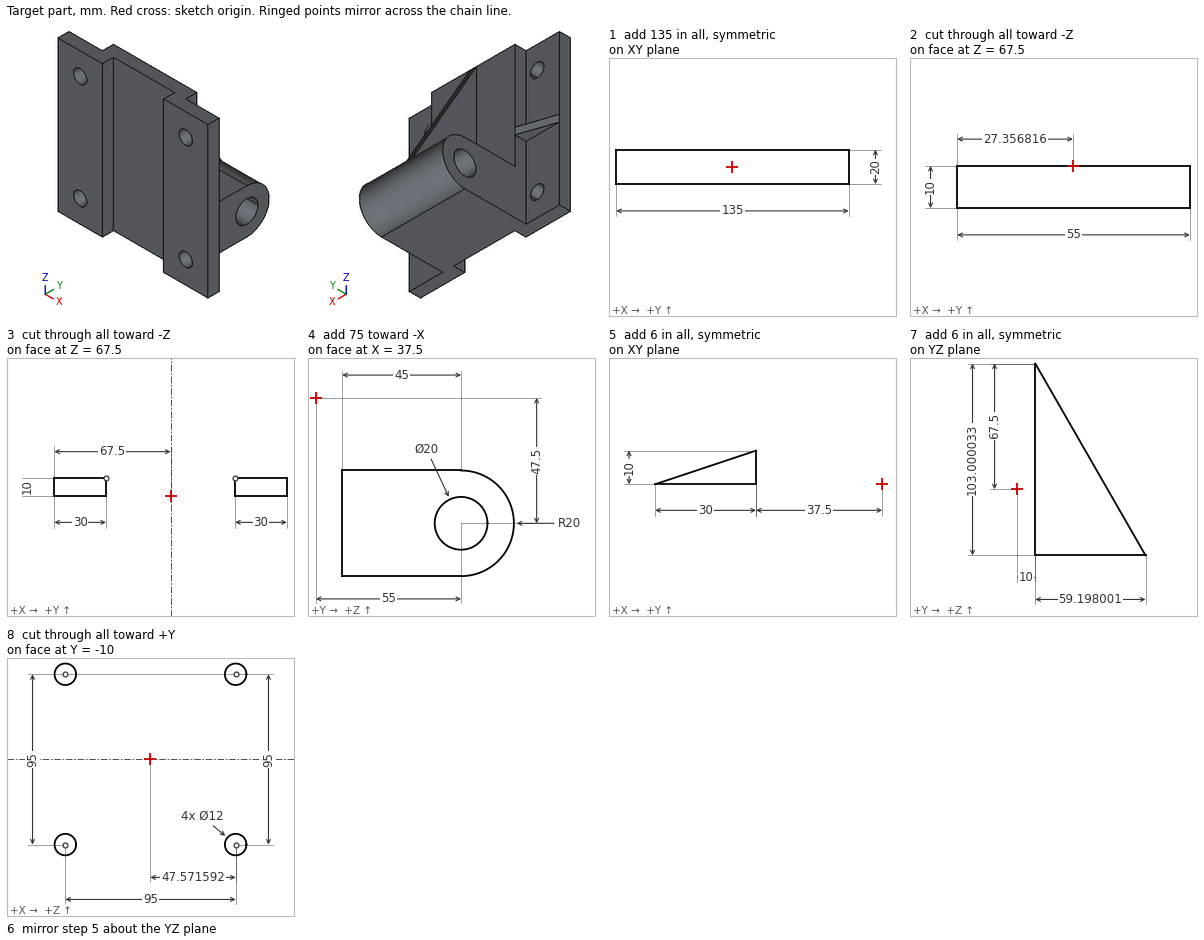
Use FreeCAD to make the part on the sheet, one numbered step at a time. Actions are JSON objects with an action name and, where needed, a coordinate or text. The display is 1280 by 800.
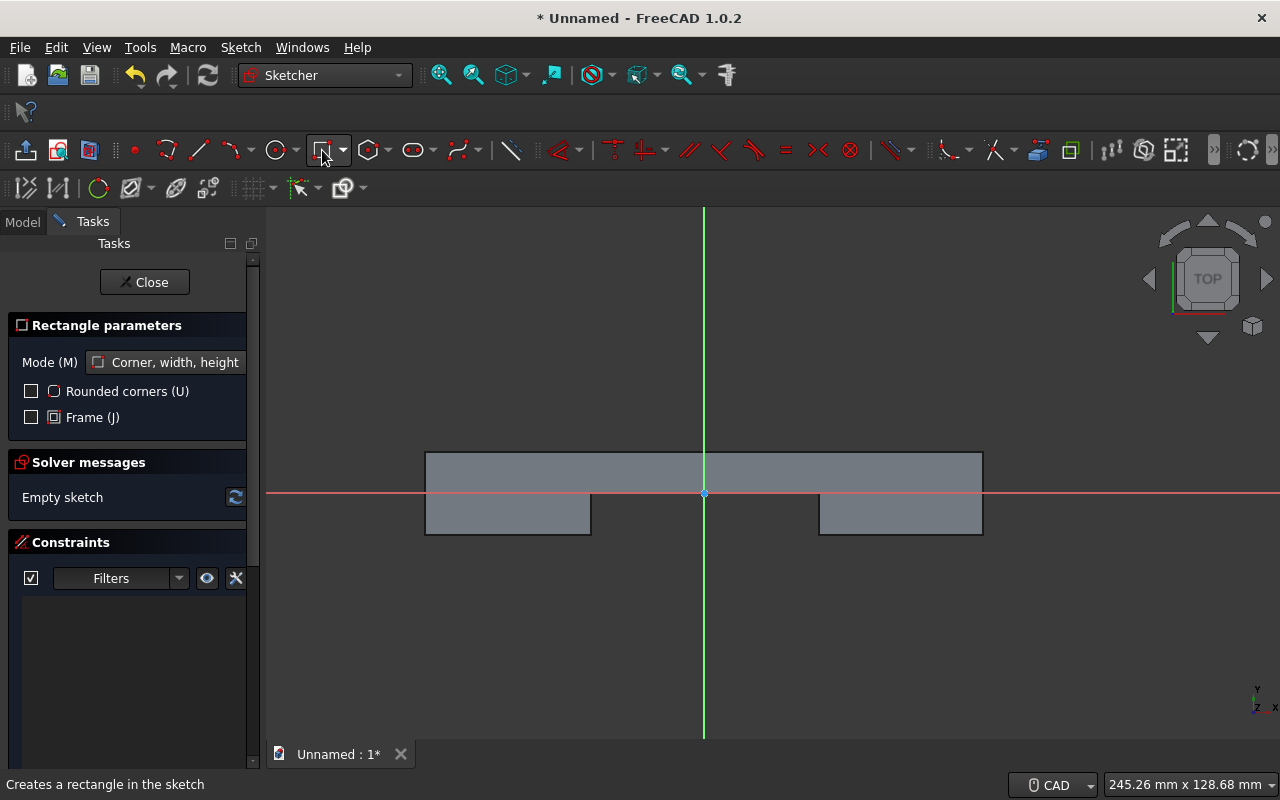
{"action": "left_click", "coordinate": [425, 452]}
{"action": "left_click", "coordinate": [549, 493]}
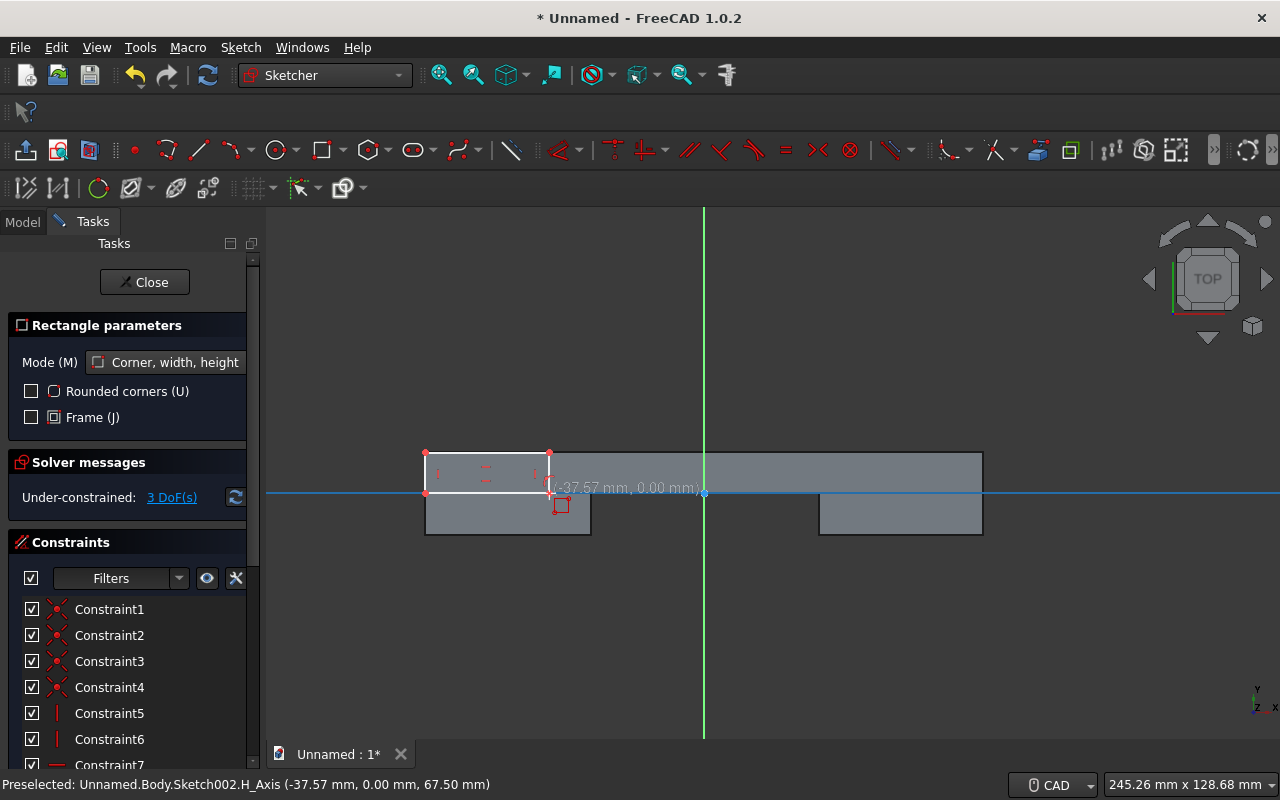
{"action": "left_click", "coordinate": [859, 452]}
{"action": "left_click", "coordinate": [983, 493]}
{"action": "key", "text": "Escape"}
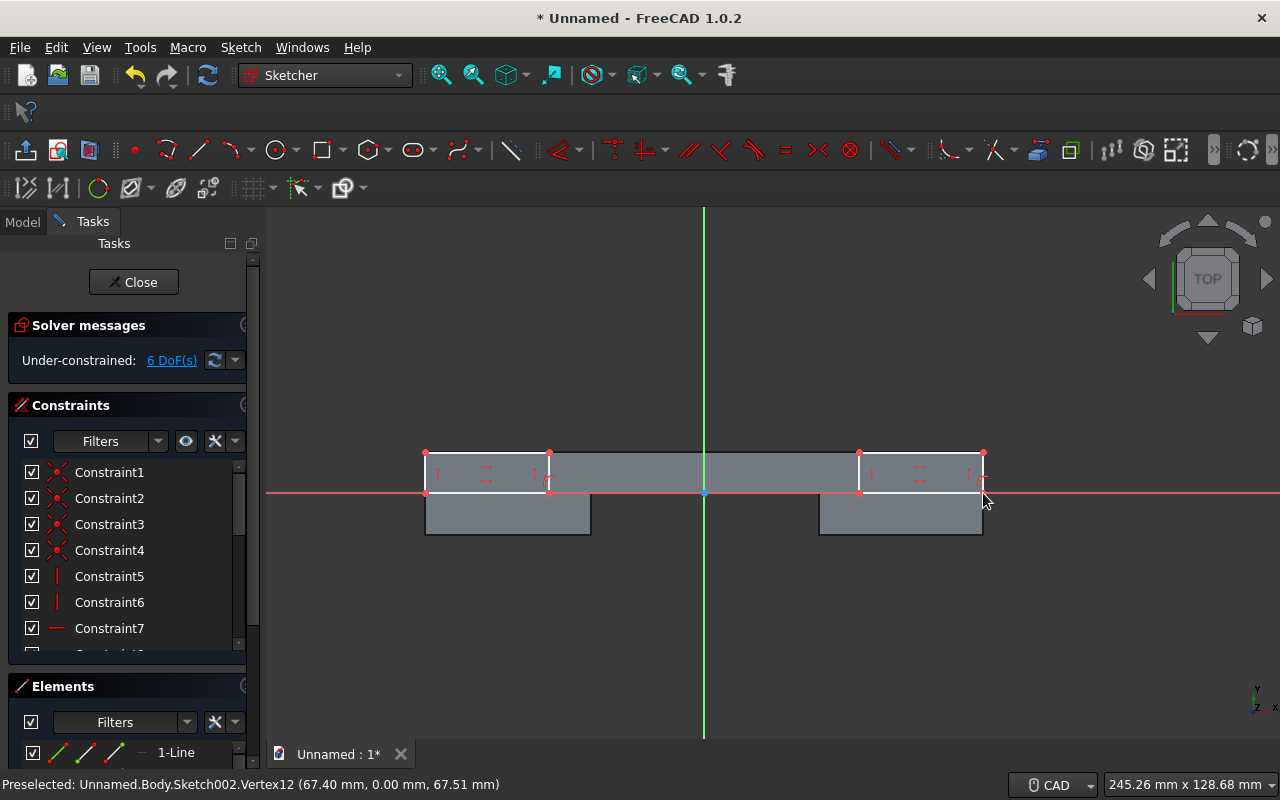
{"action": "left_click", "coordinate": [549, 453]}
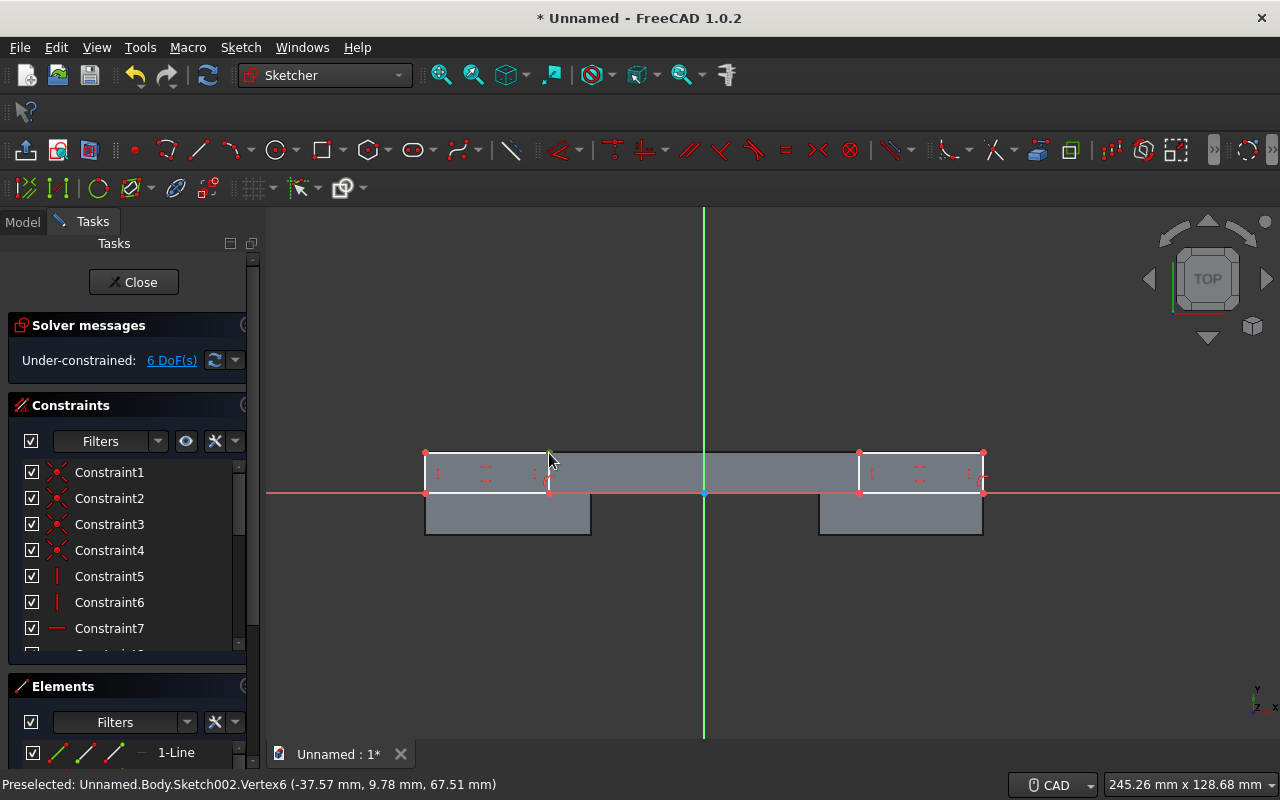
{"action": "left_click", "coordinate": [859, 453]}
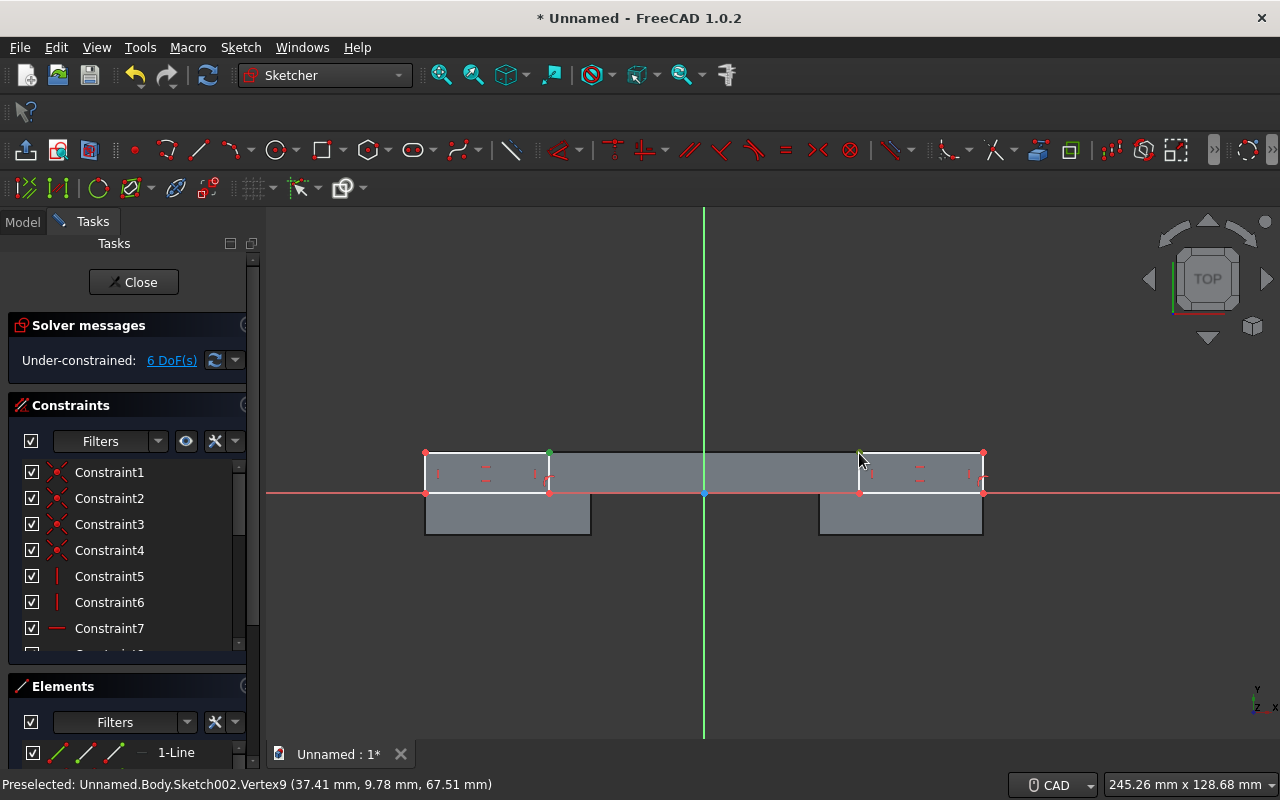
{"action": "left_click", "coordinate": [704, 677]}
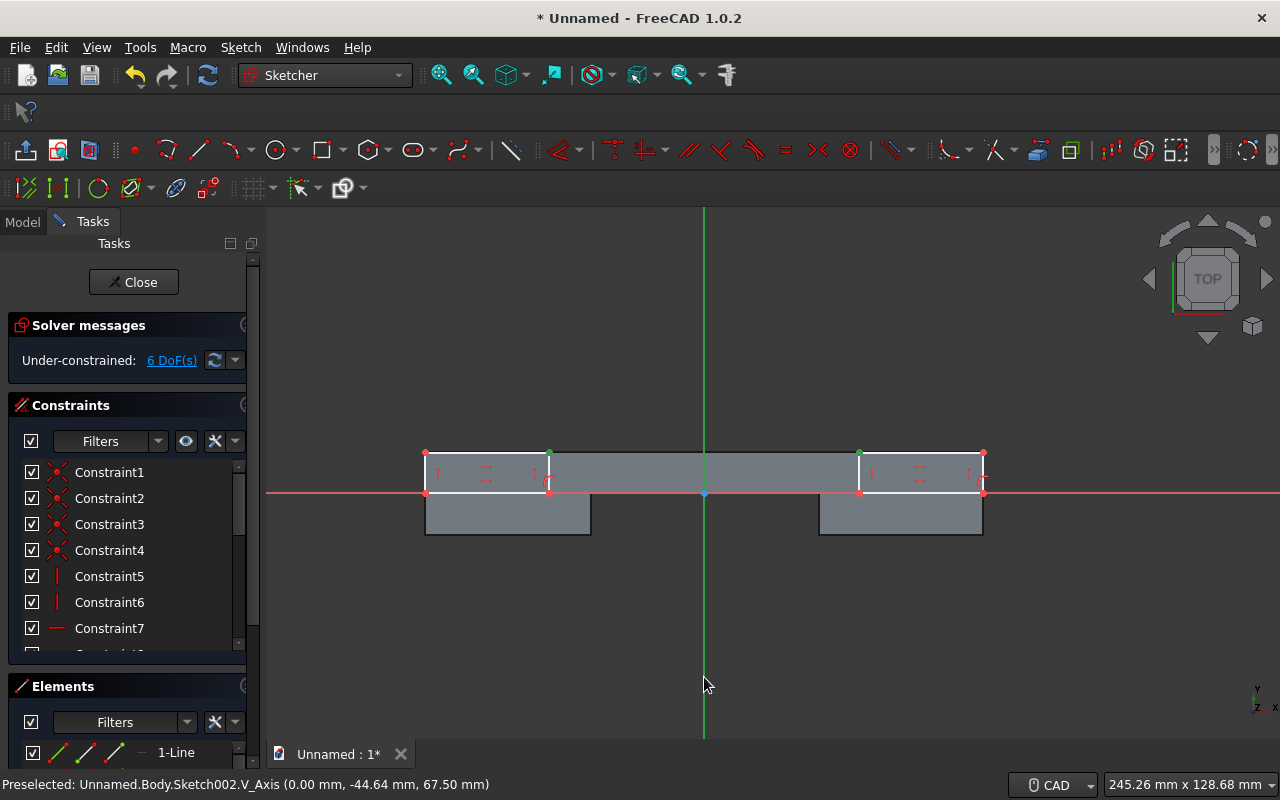
{"action": "left_click", "coordinate": [818, 150]}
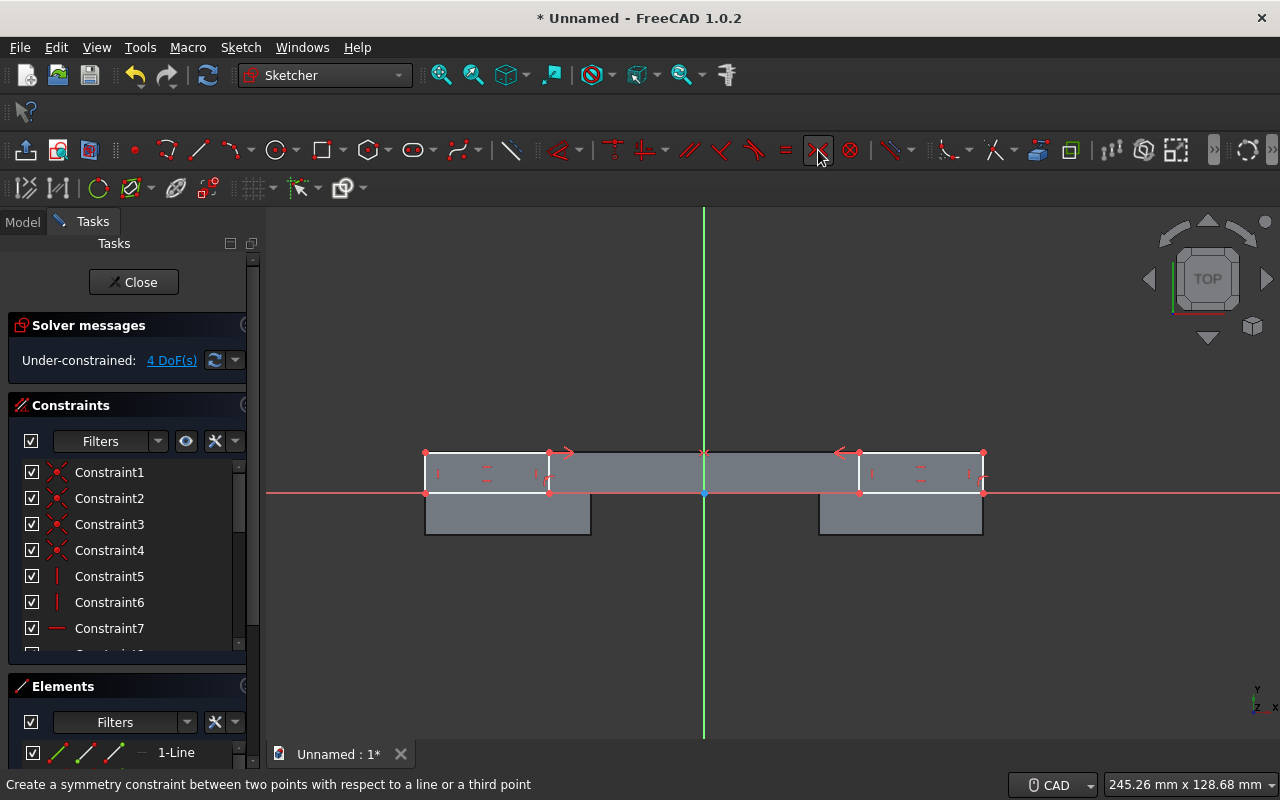
{"action": "key", "text": "d"}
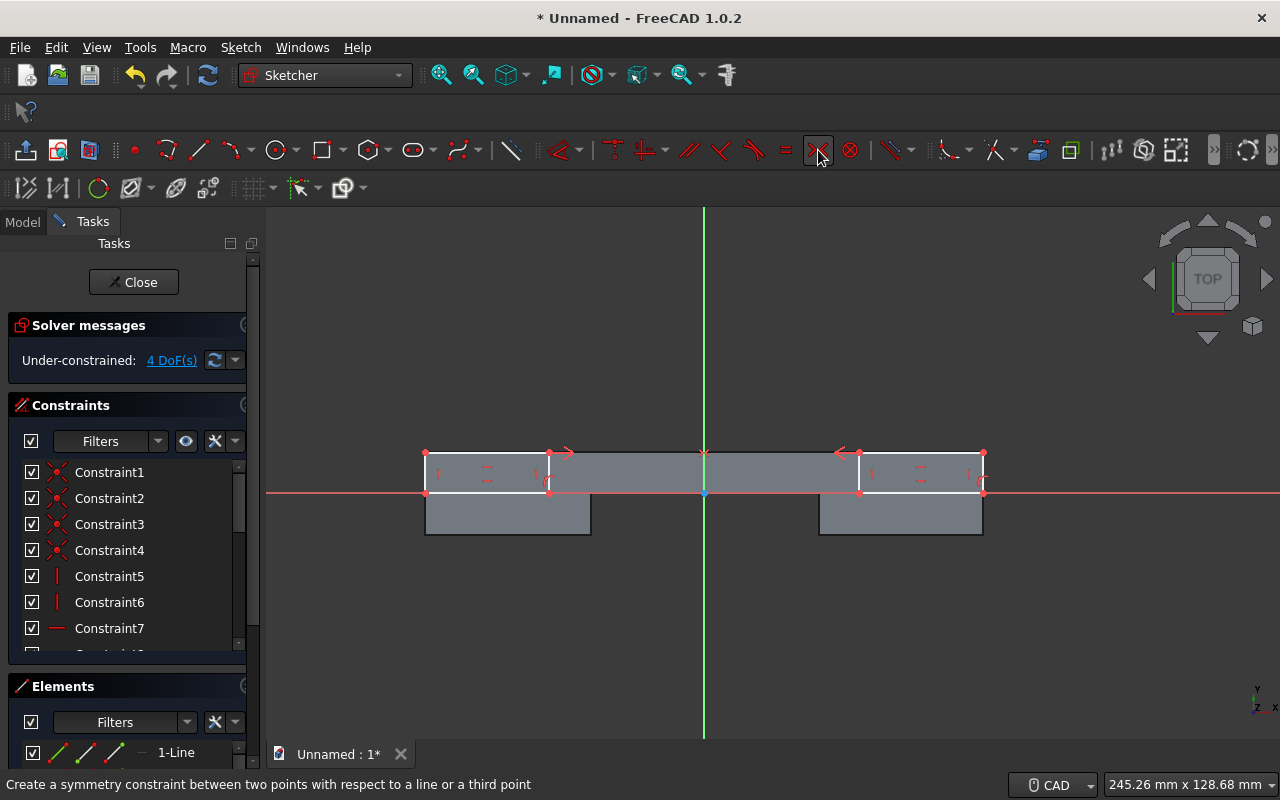
{"action": "left_click", "coordinate": [425, 465]}
{"action": "left_click", "coordinate": [391, 473]}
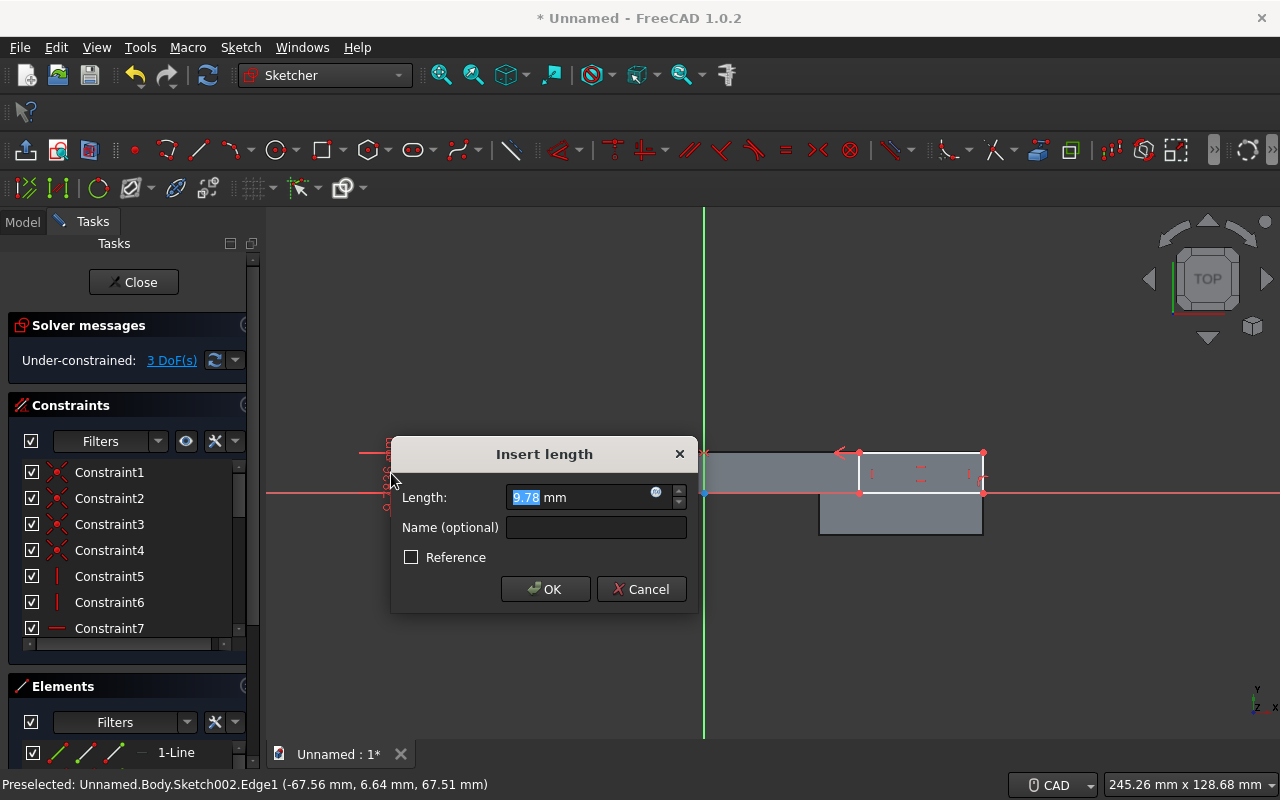
{"action": "type", "text": "10"}
{"action": "key", "text": "Return"}